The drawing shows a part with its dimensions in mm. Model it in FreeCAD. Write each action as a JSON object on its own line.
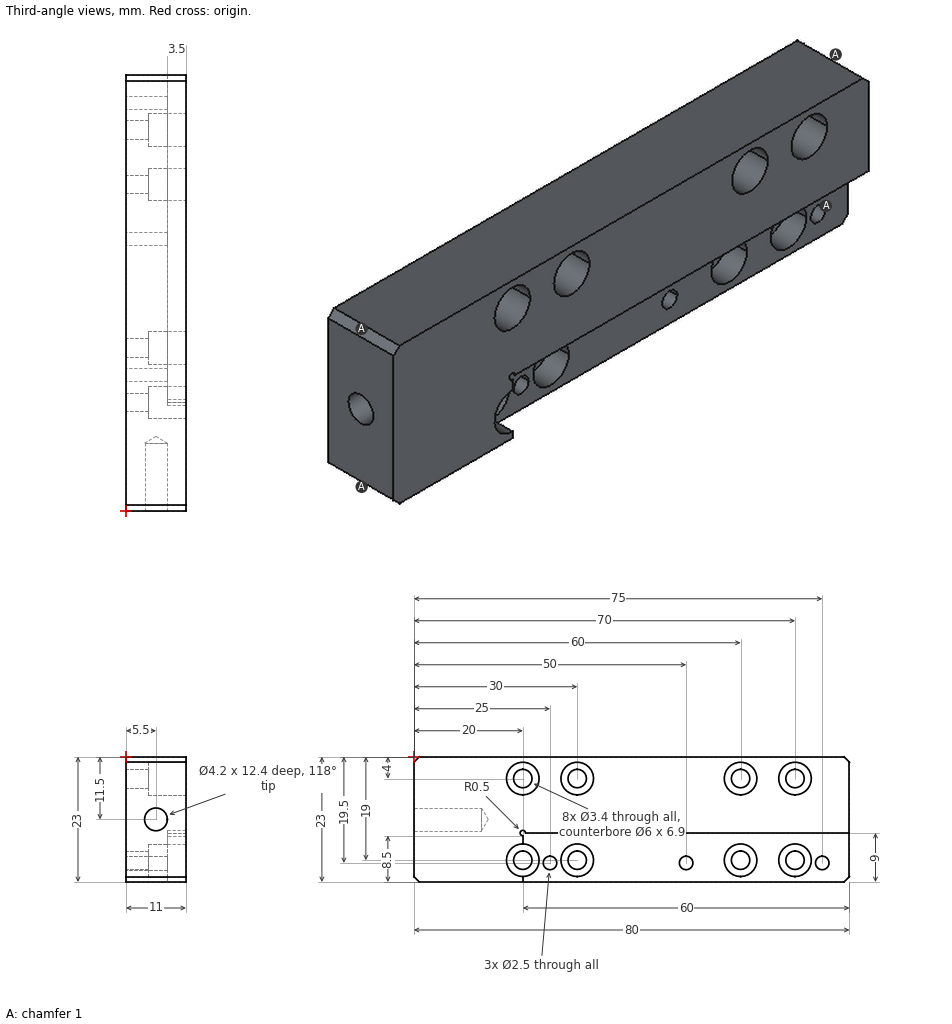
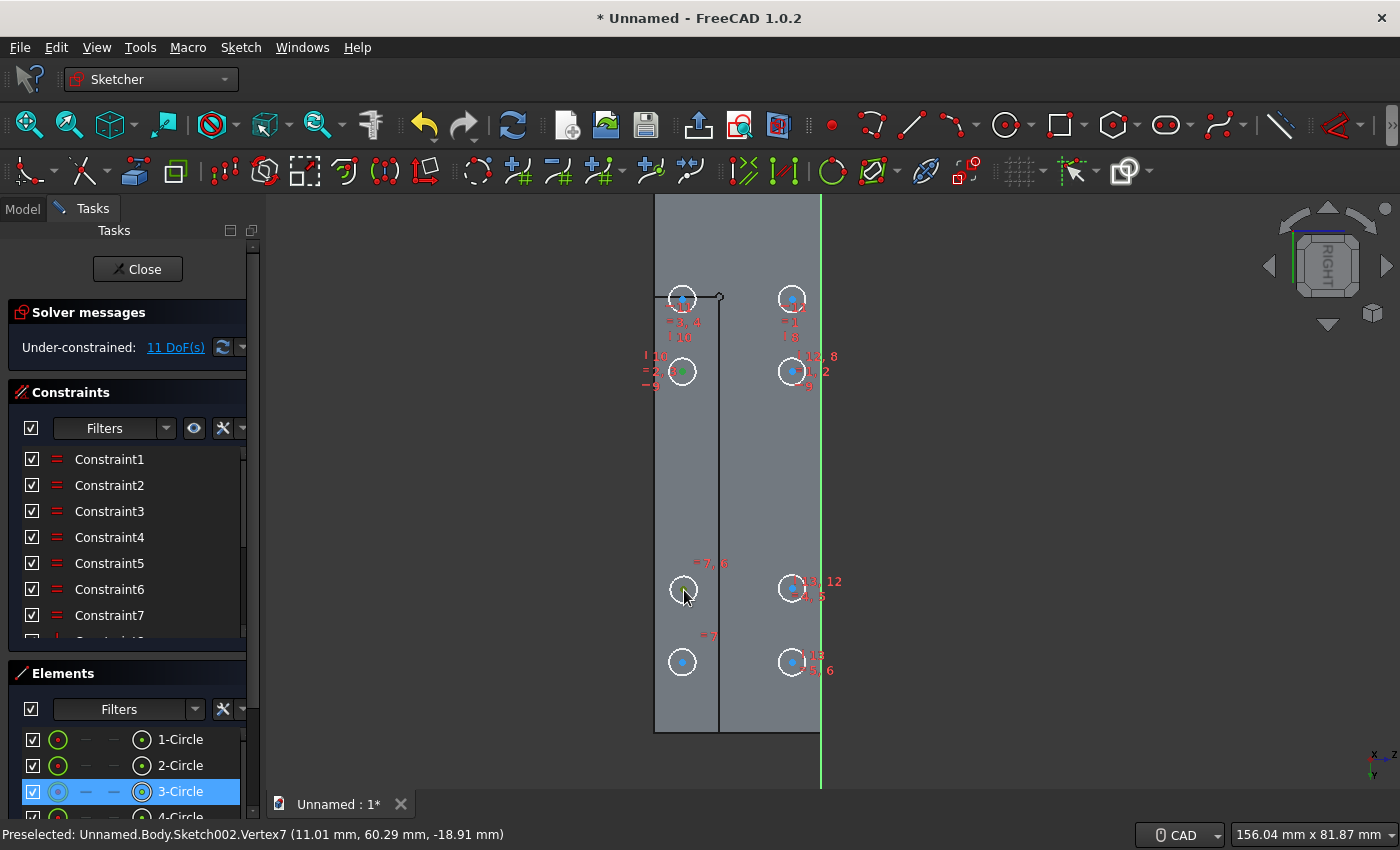
{"action": "key", "text": "v"}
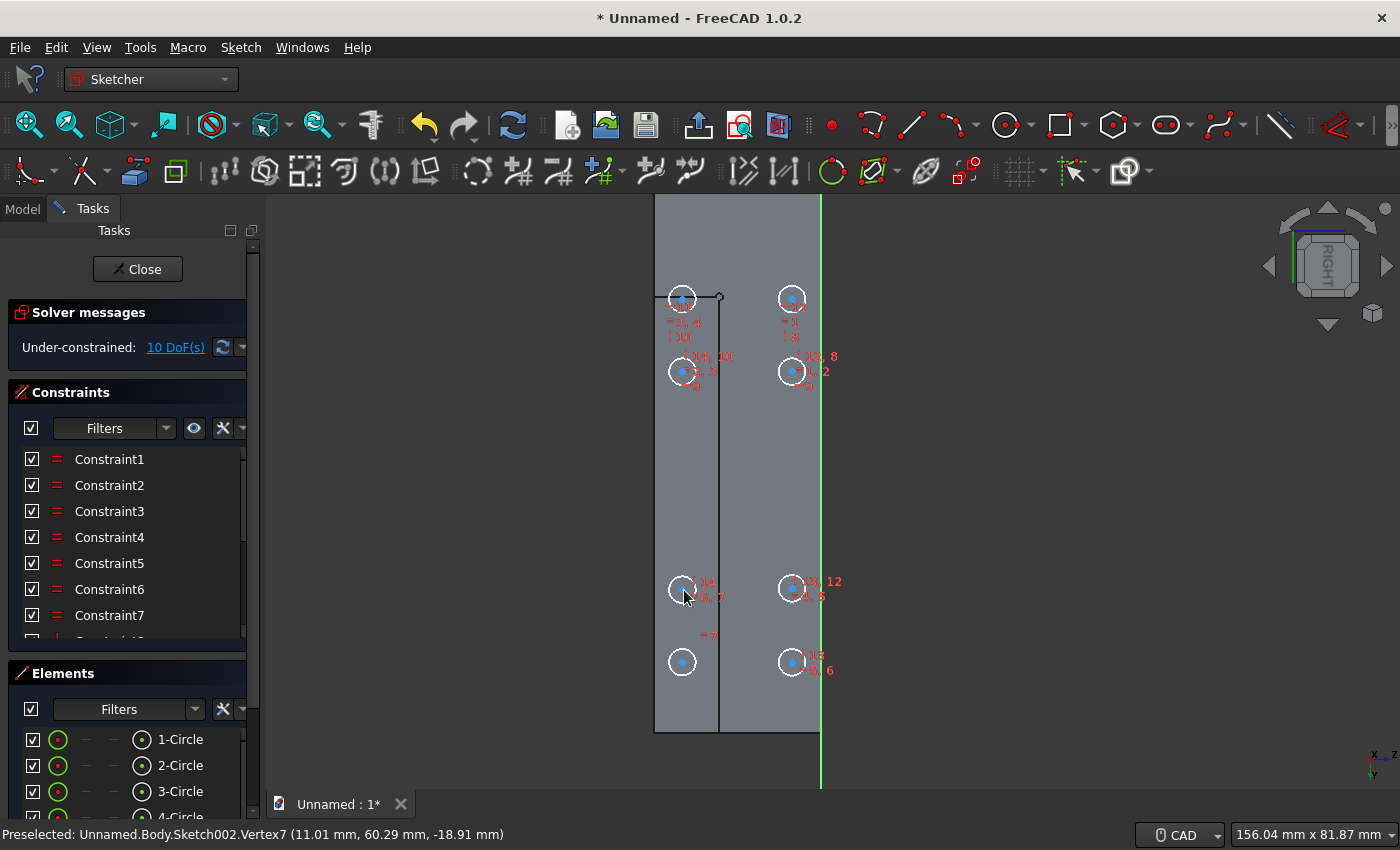
{"action": "left_click", "coordinate": [792, 588]}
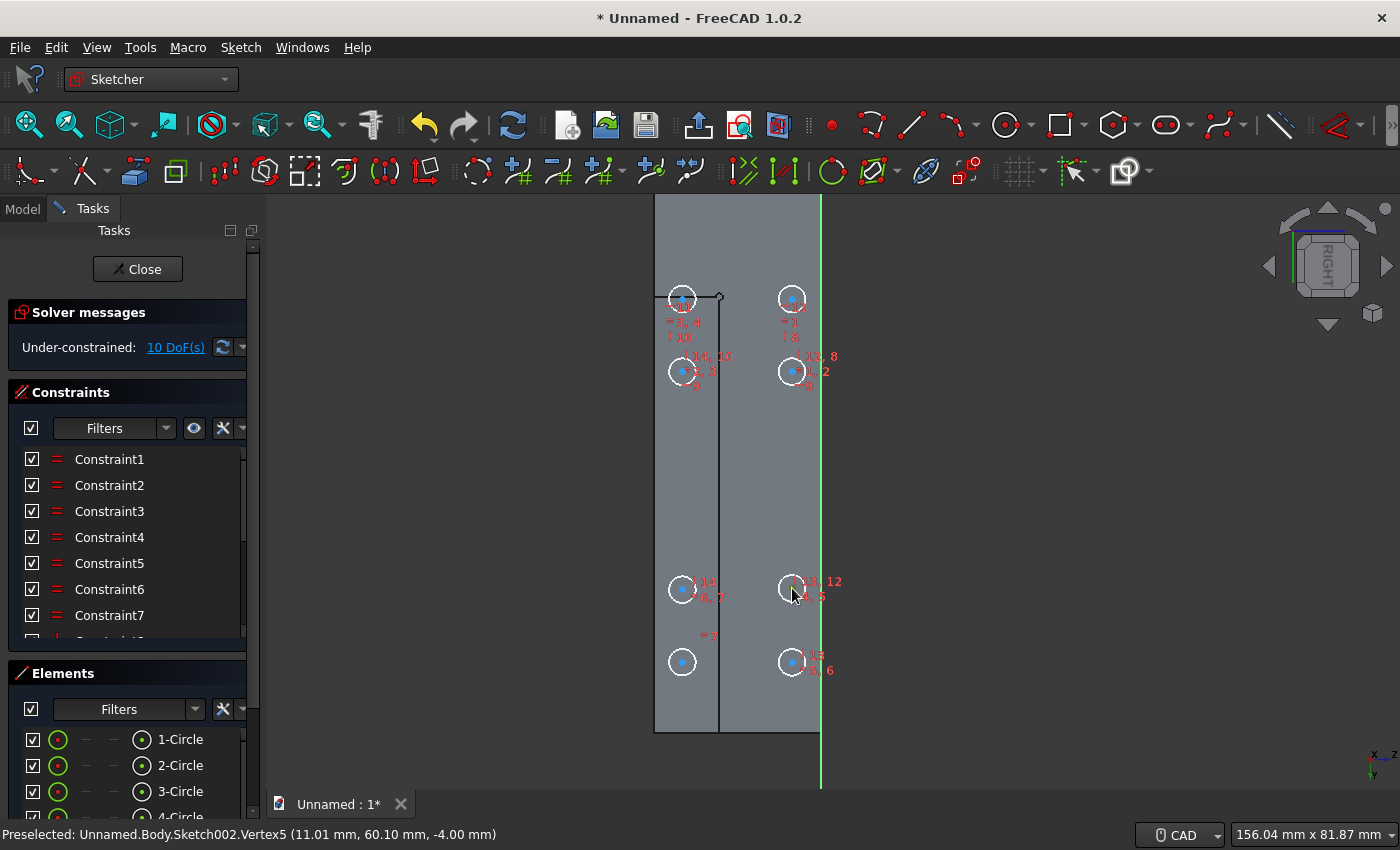
{"action": "left_click", "coordinate": [682, 590]}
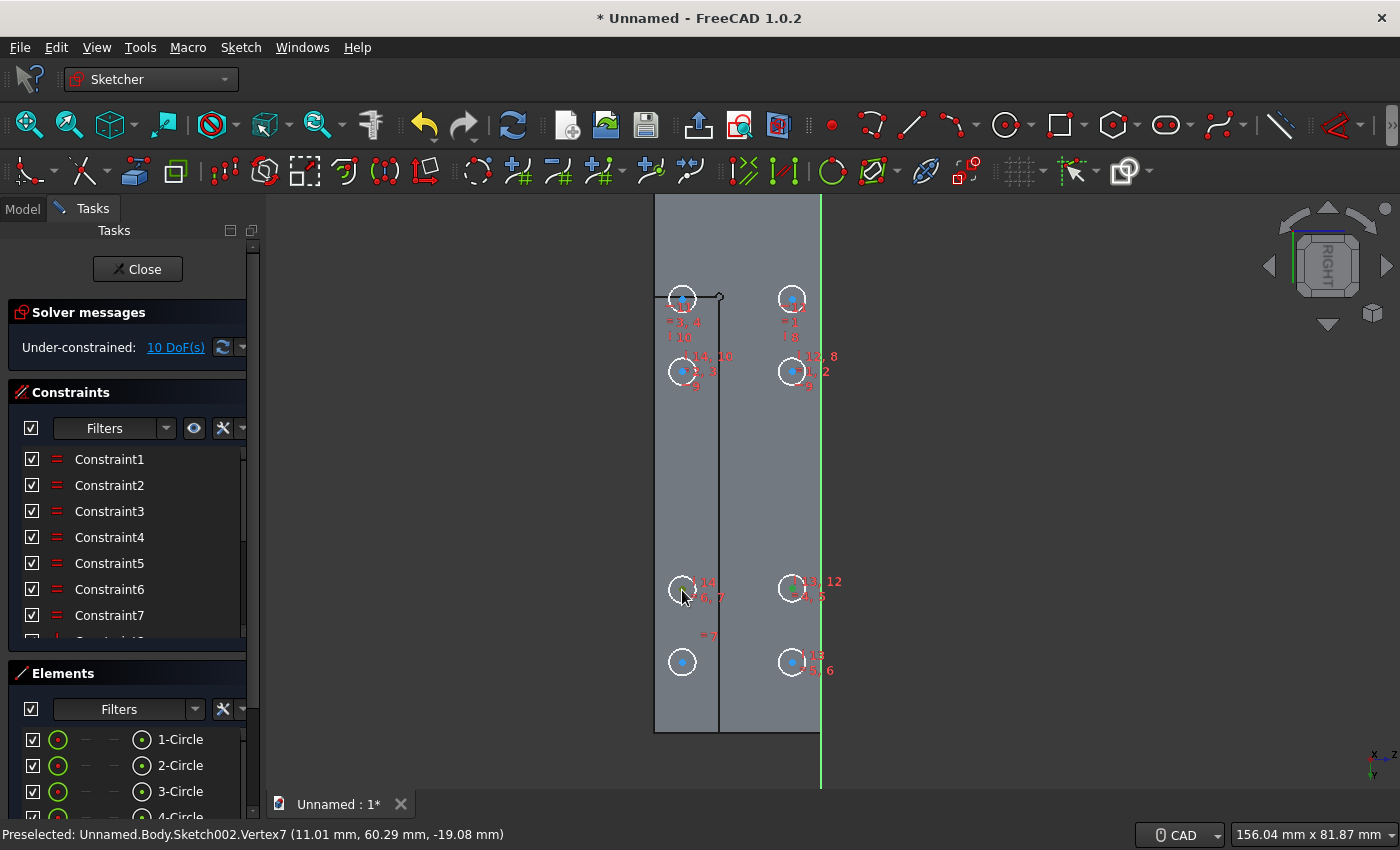
{"action": "key", "text": "h"}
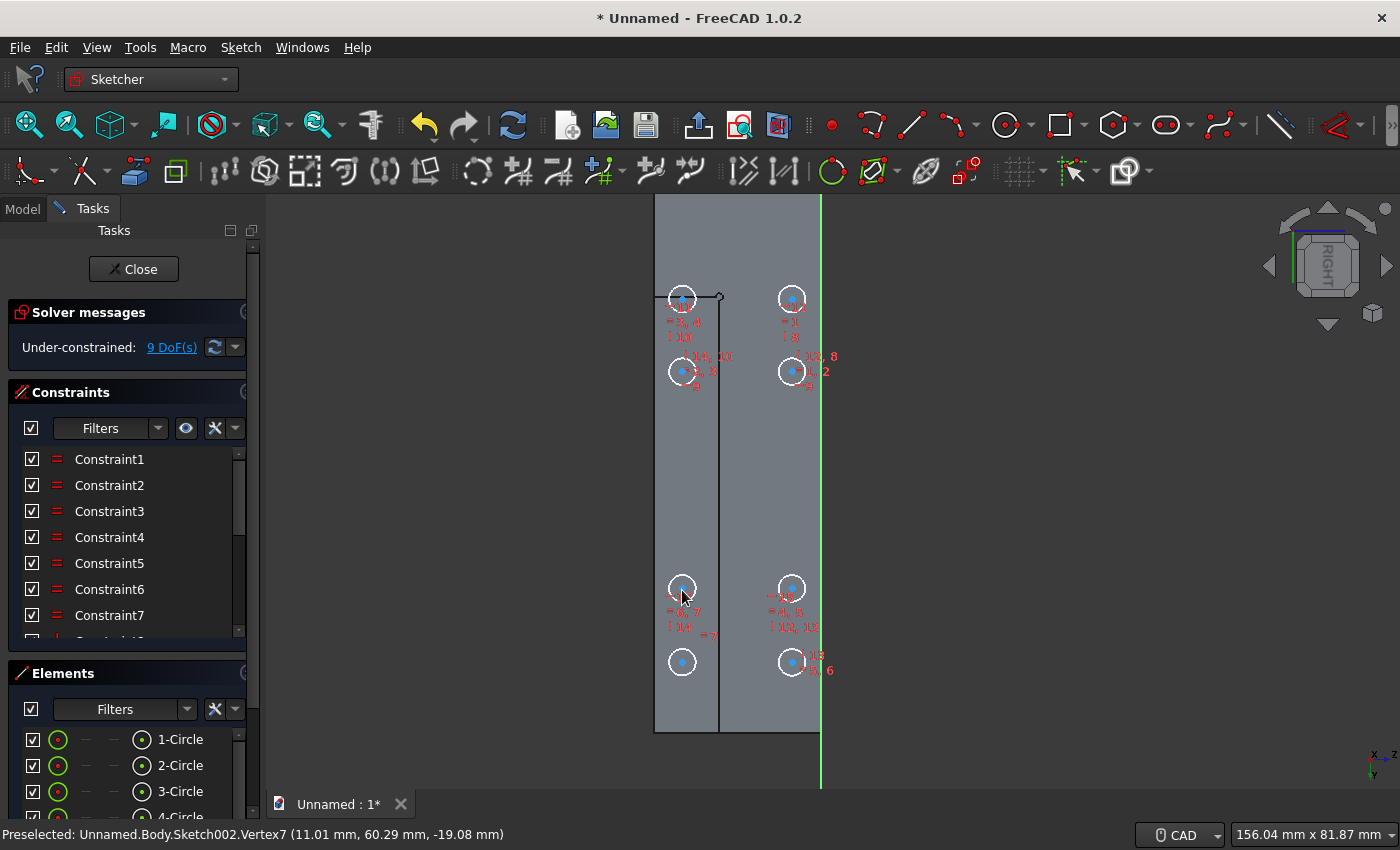
{"action": "left_click", "coordinate": [682, 588]}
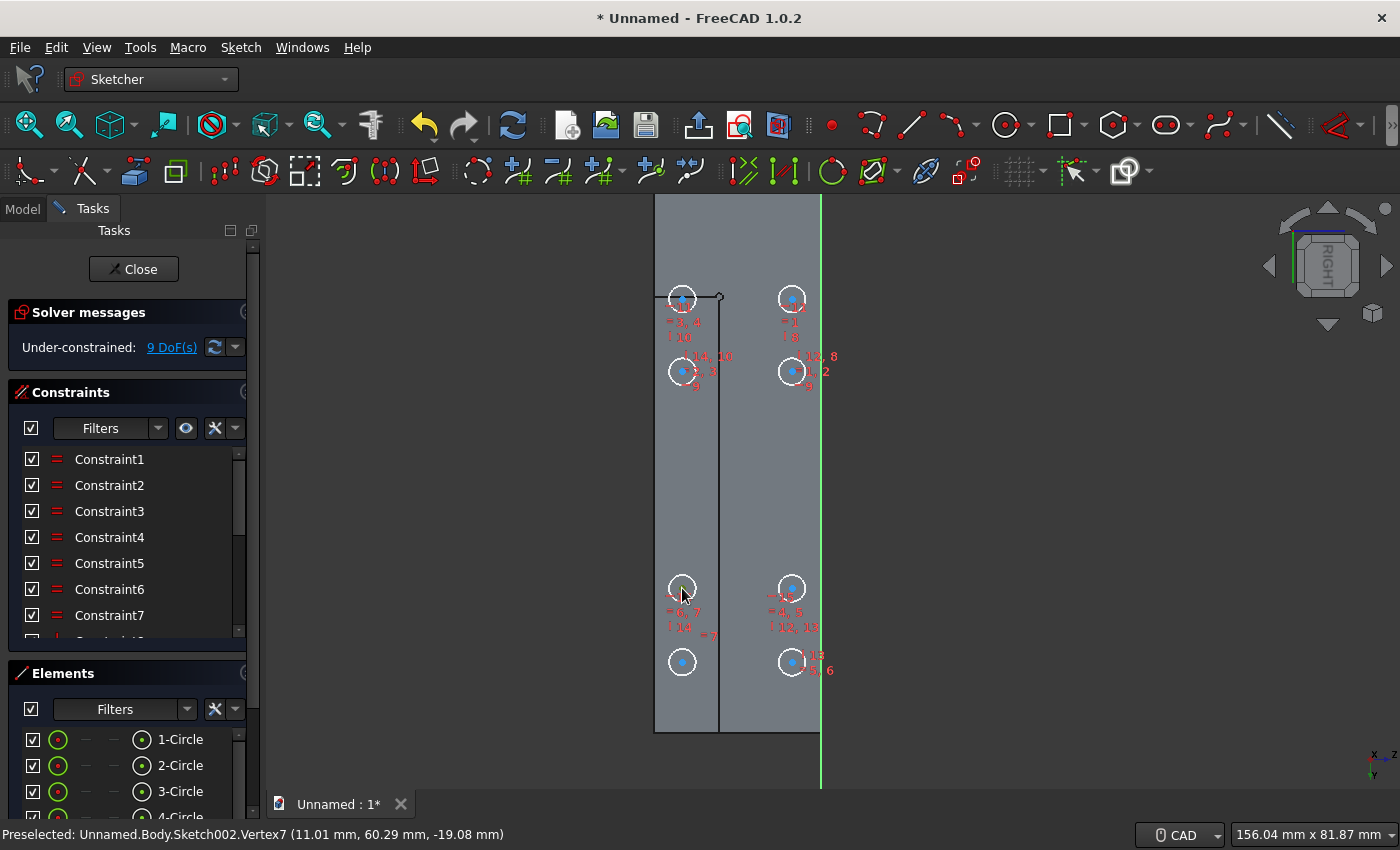
{"action": "left_click", "coordinate": [682, 662]}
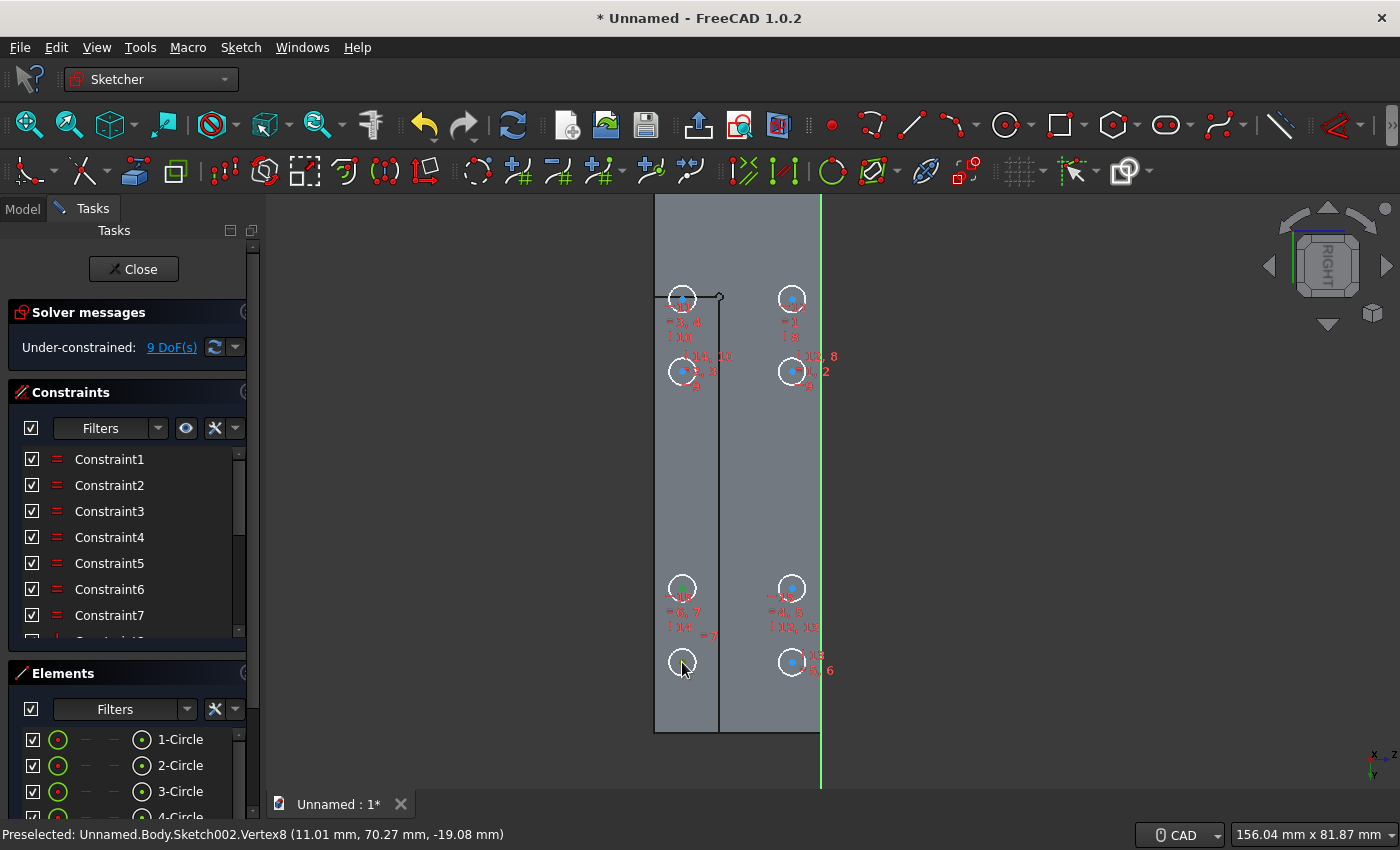
{"action": "key", "text": "v"}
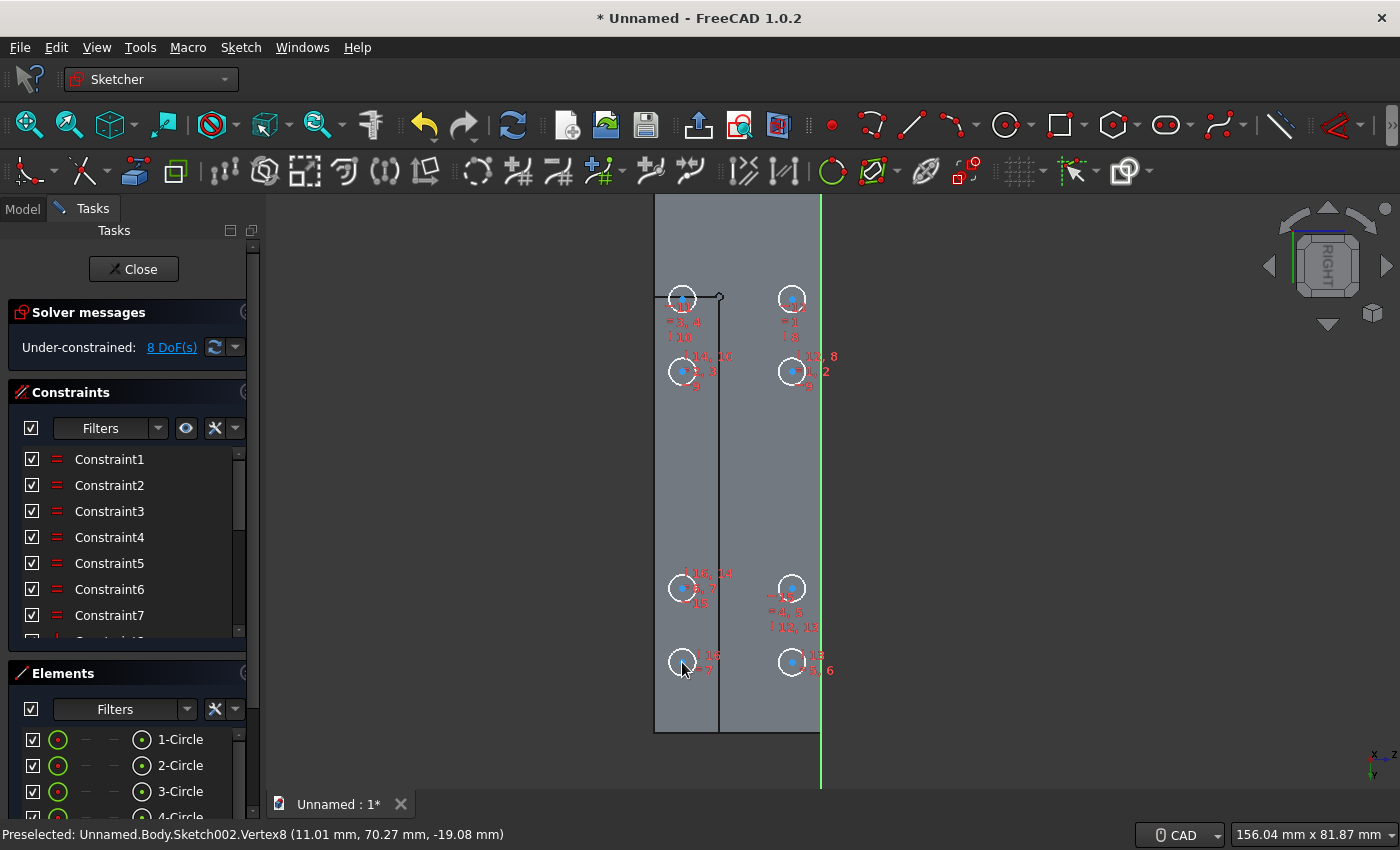
{"action": "left_click", "coordinate": [792, 662]}